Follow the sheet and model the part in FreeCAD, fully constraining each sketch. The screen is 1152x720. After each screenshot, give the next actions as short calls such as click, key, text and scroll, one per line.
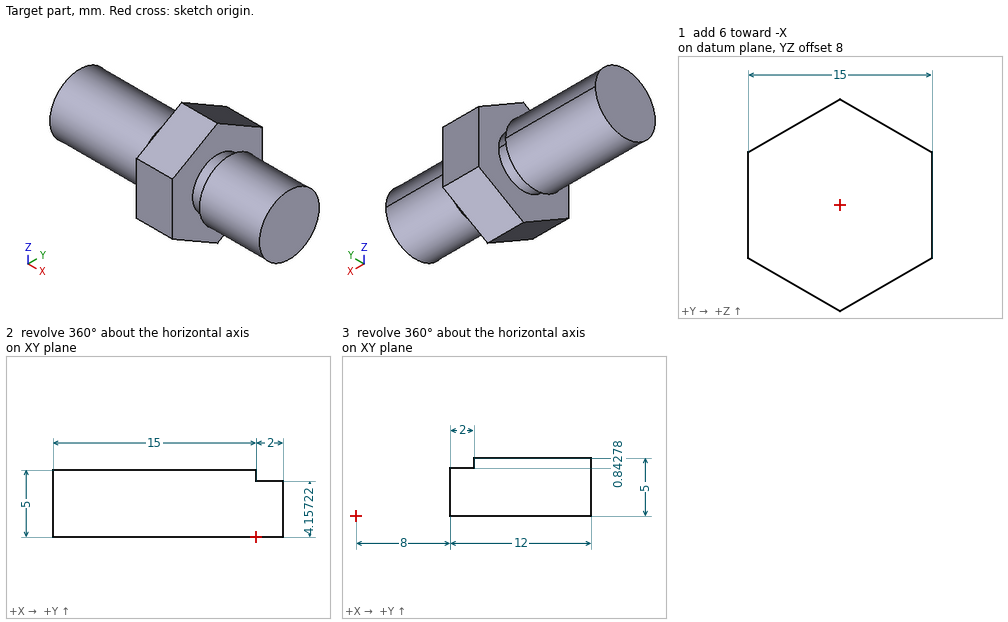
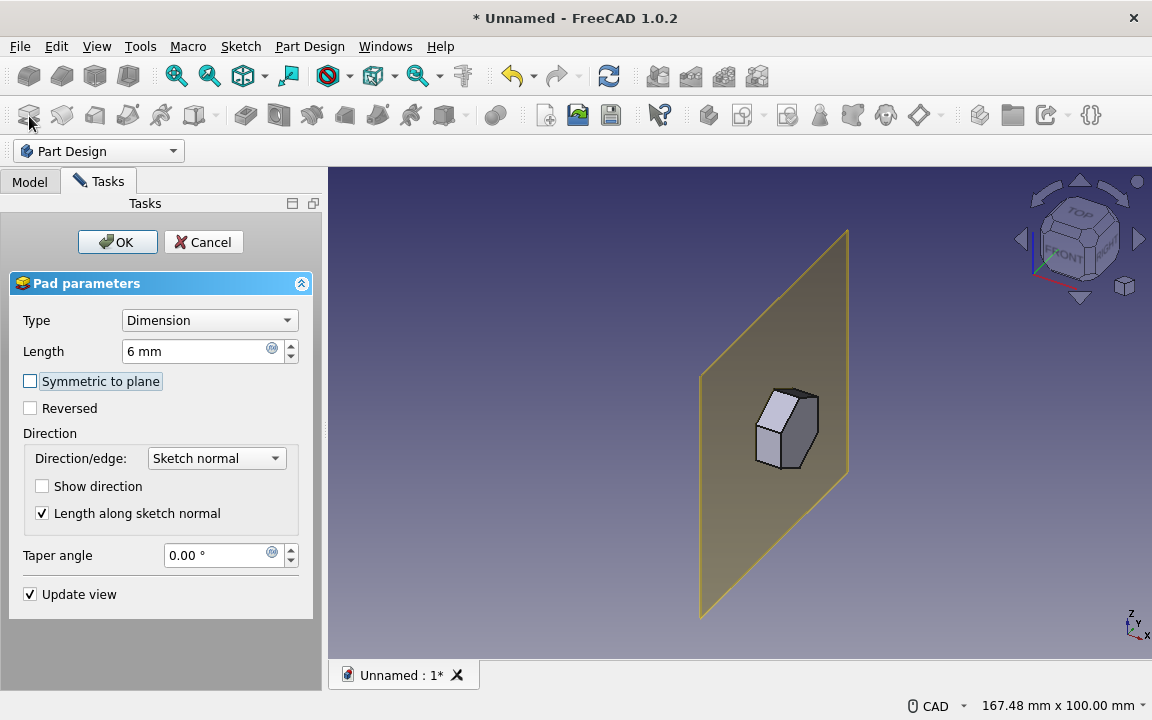
click(31, 408)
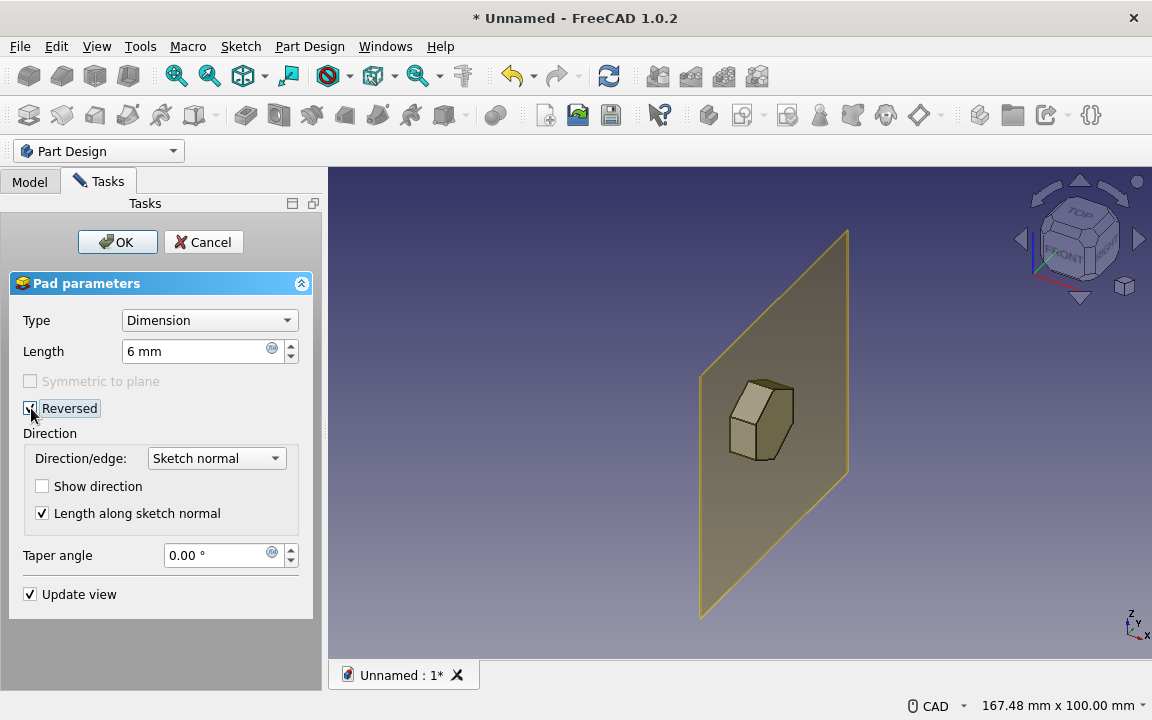
click(118, 242)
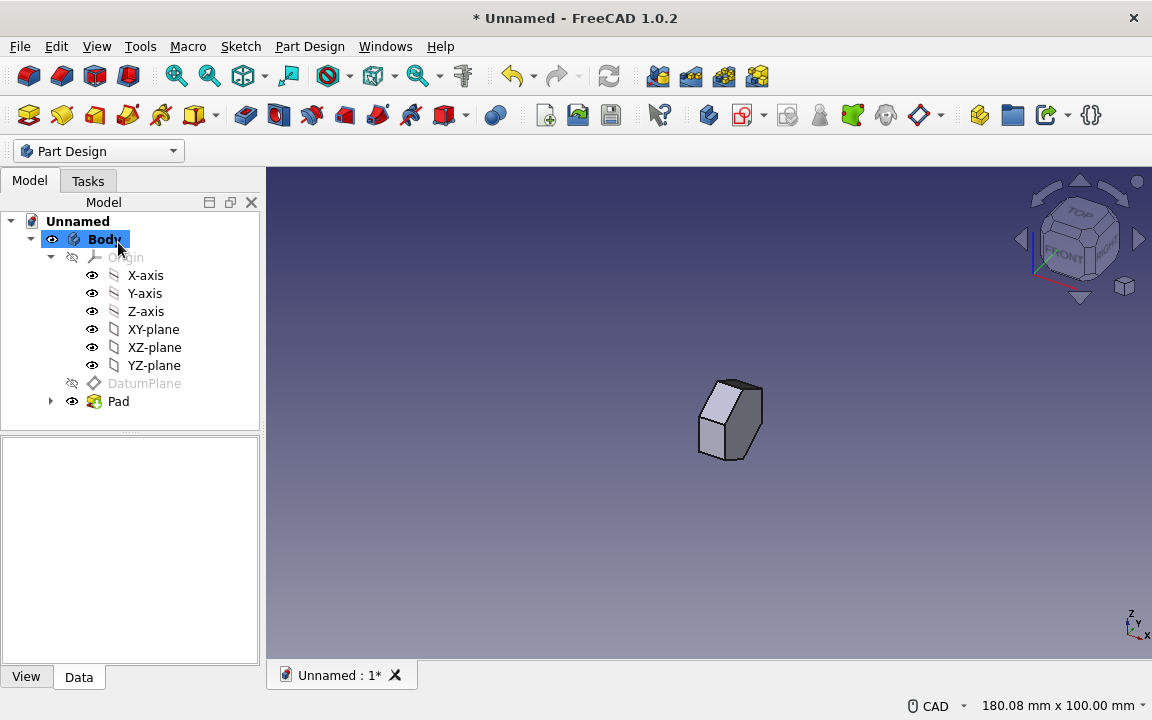
click(177, 76)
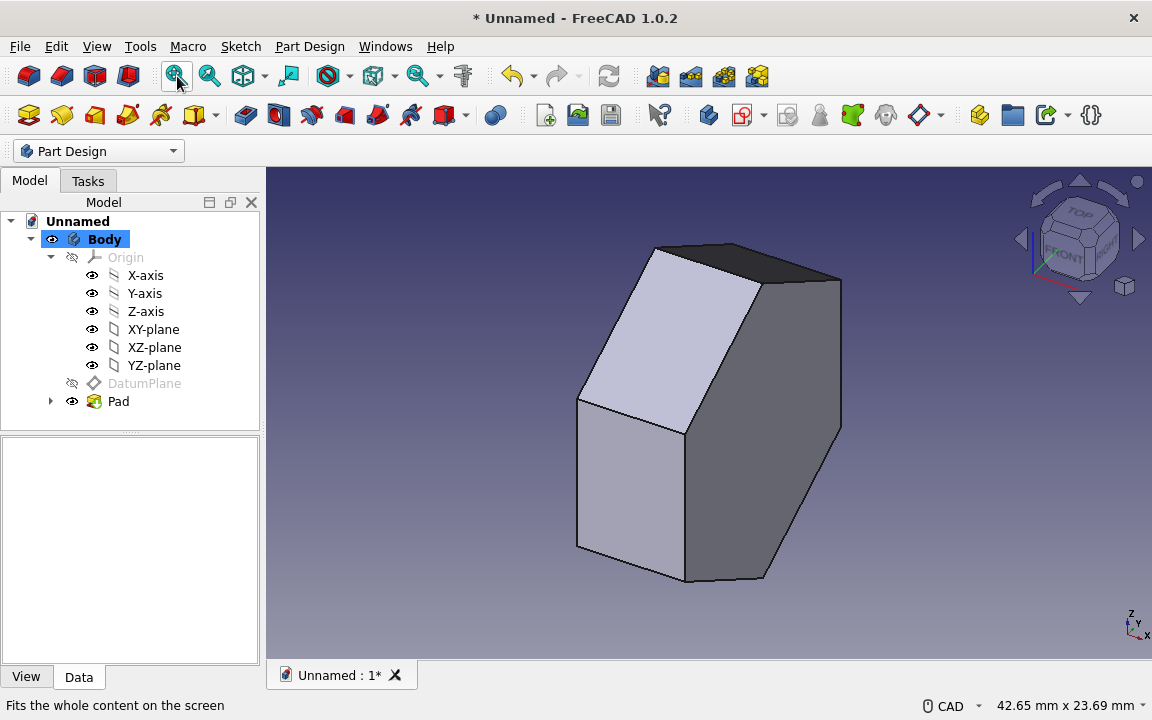
click(742, 116)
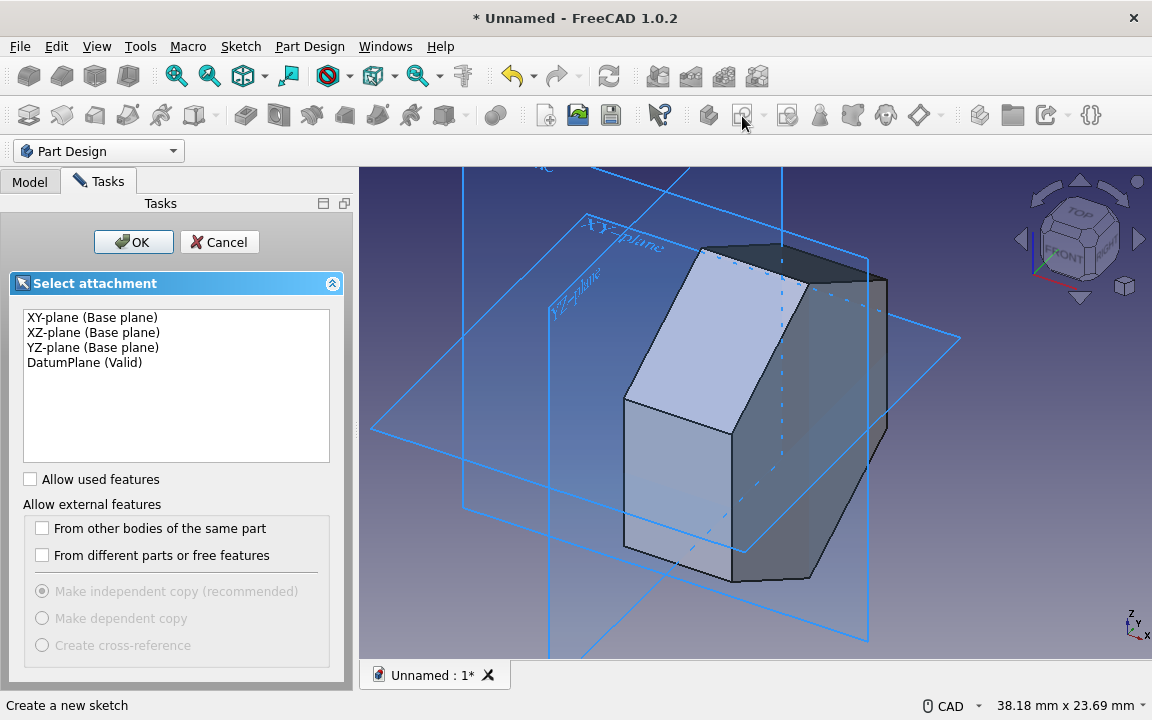
click(84, 318)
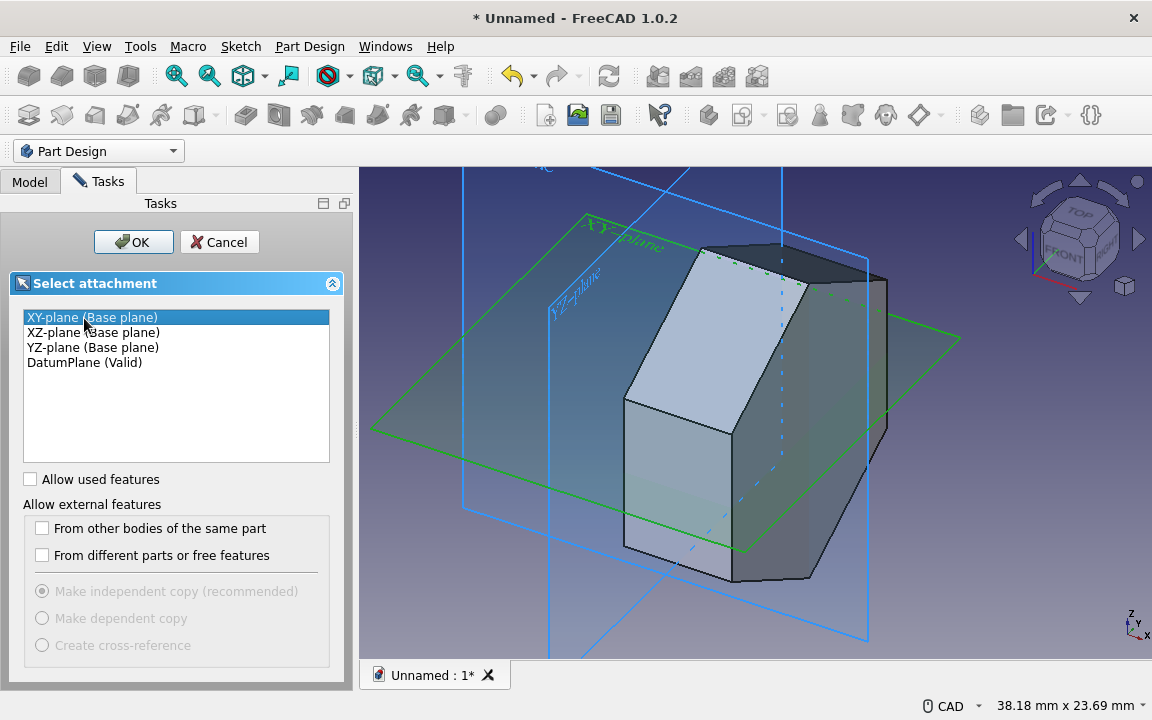
click(134, 242)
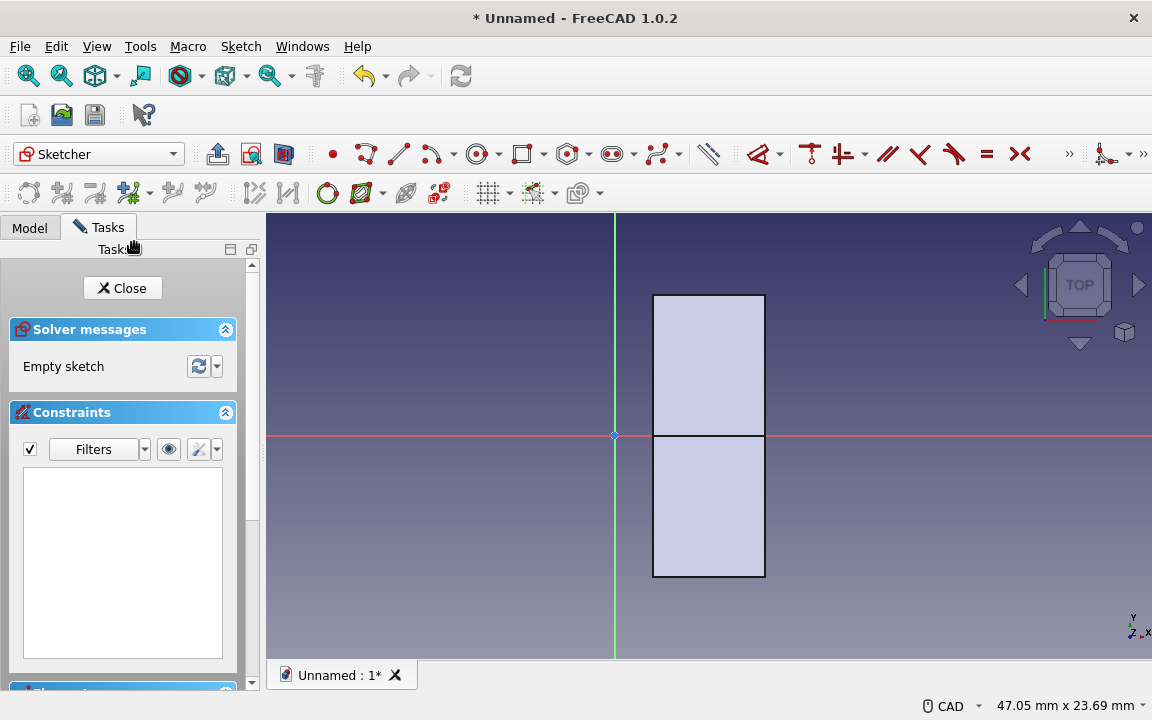
click(284, 154)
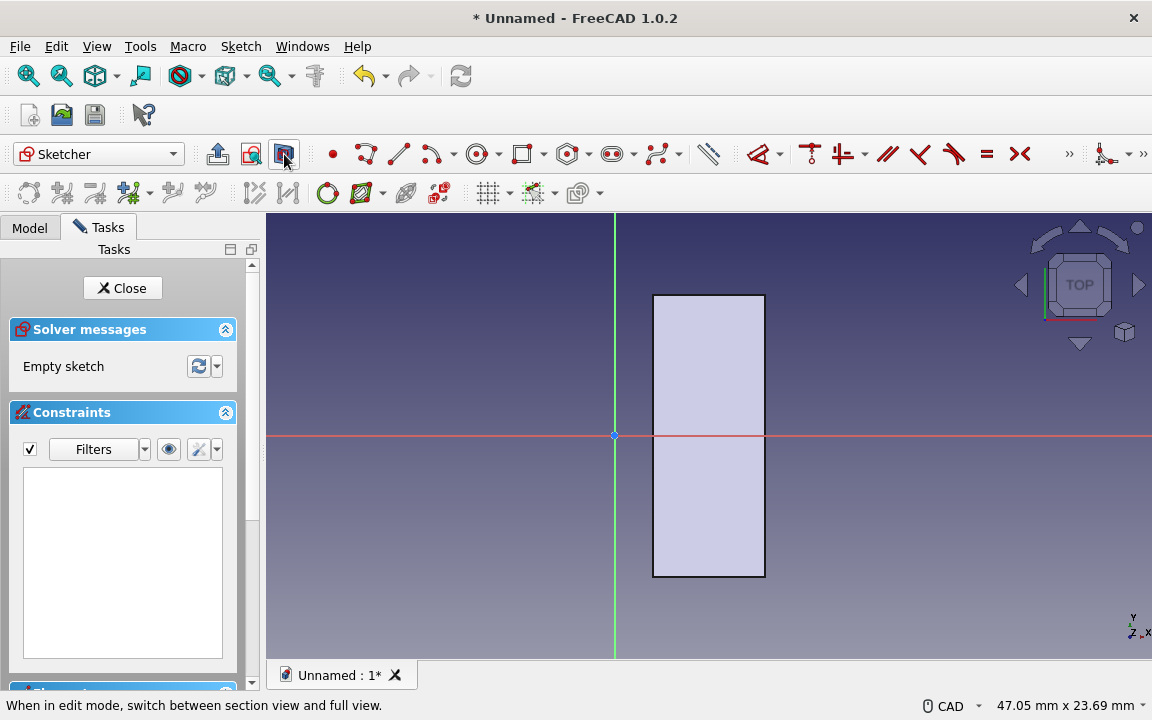
scroll(294, 293, up, 2)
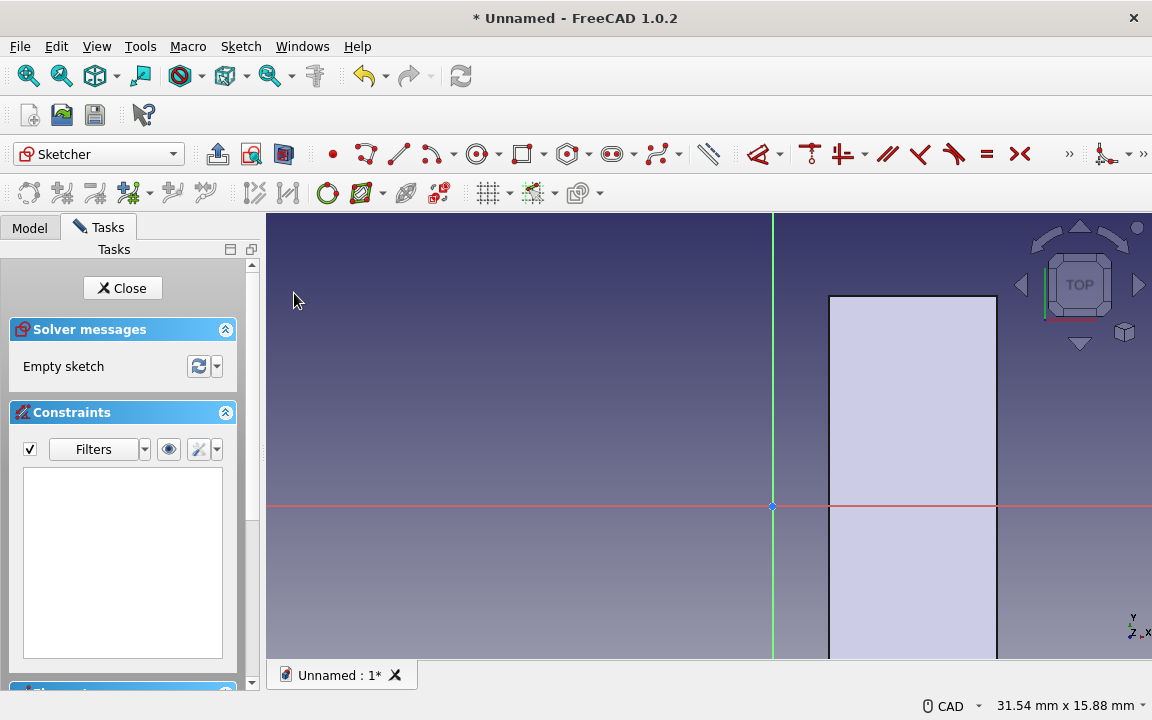
click(366, 154)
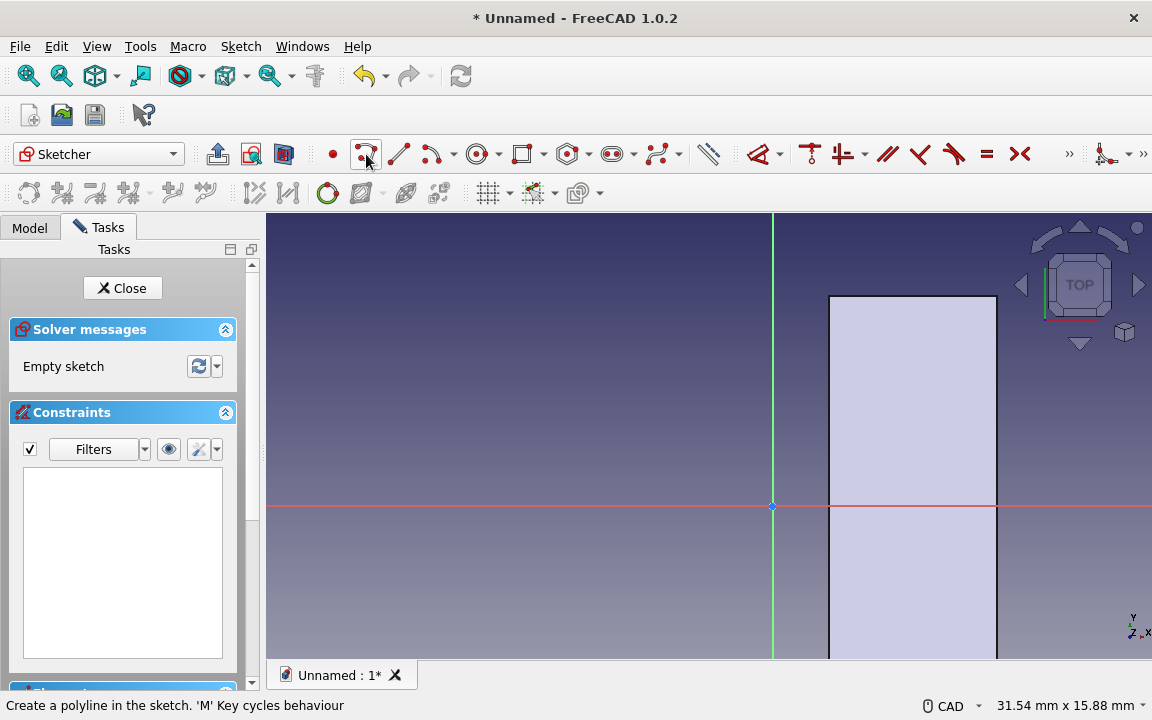
click(829, 506)
click(829, 389)
click(773, 389)
click(764, 366)
click(351, 366)
click(351, 497)
click(829, 506)
key(Escape)
key(Escape)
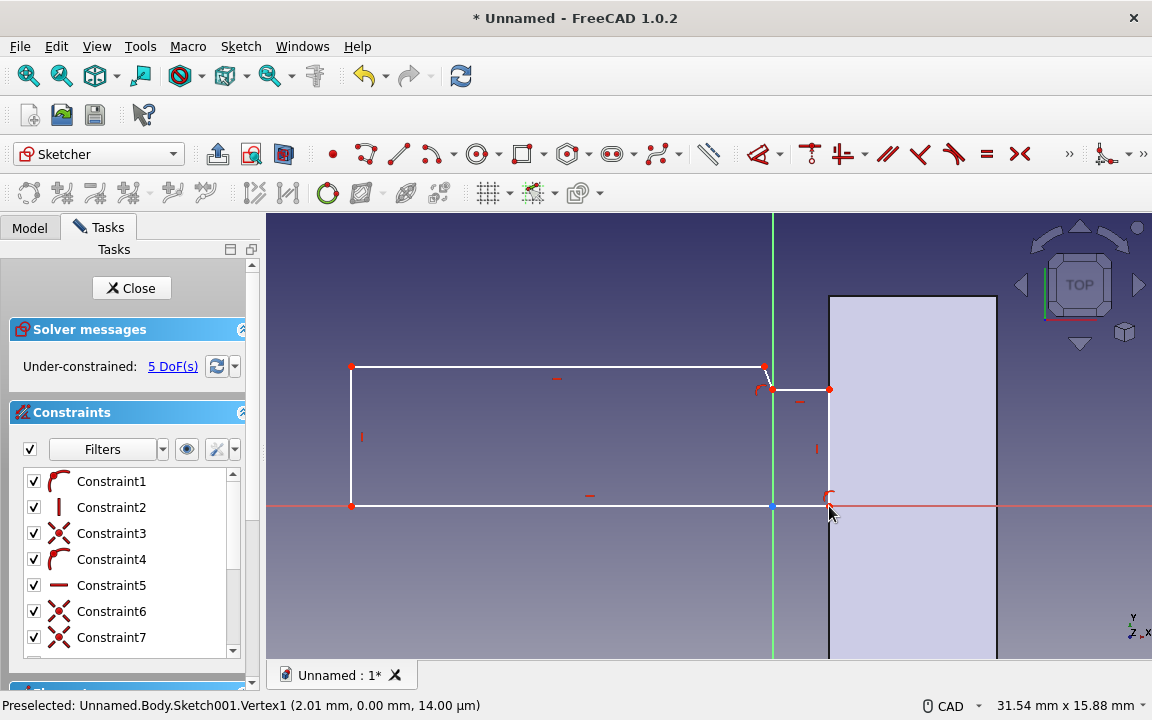
scroll(769, 381, up, 2)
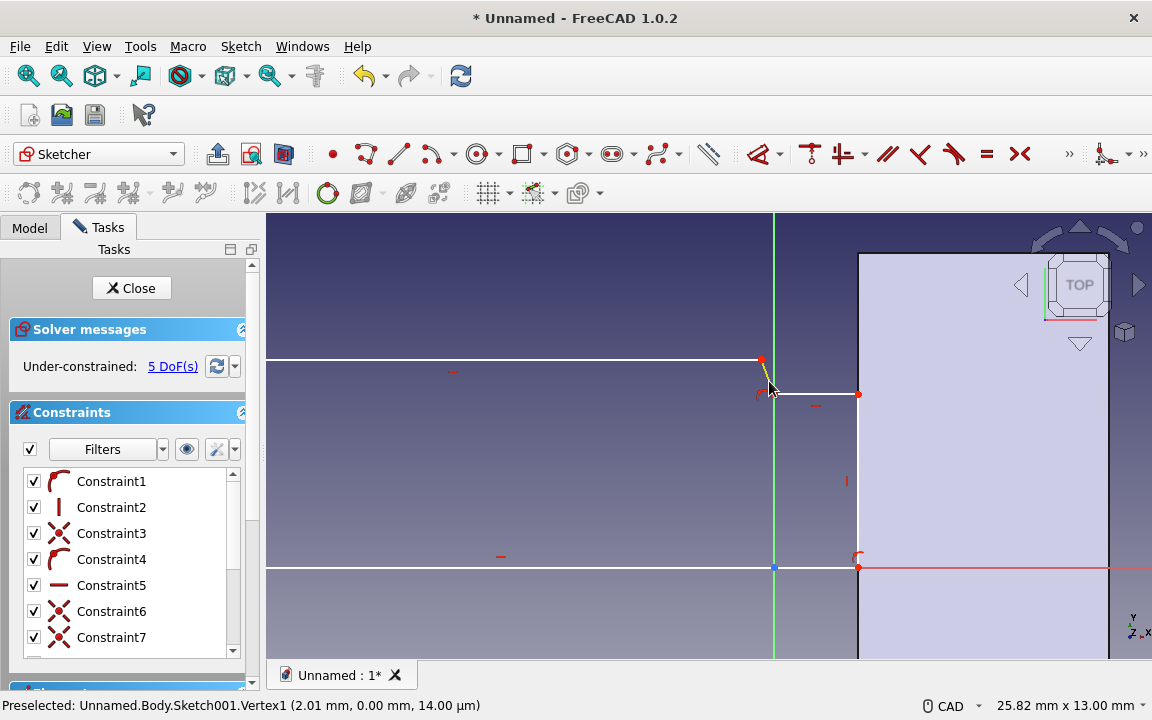
click(769, 381)